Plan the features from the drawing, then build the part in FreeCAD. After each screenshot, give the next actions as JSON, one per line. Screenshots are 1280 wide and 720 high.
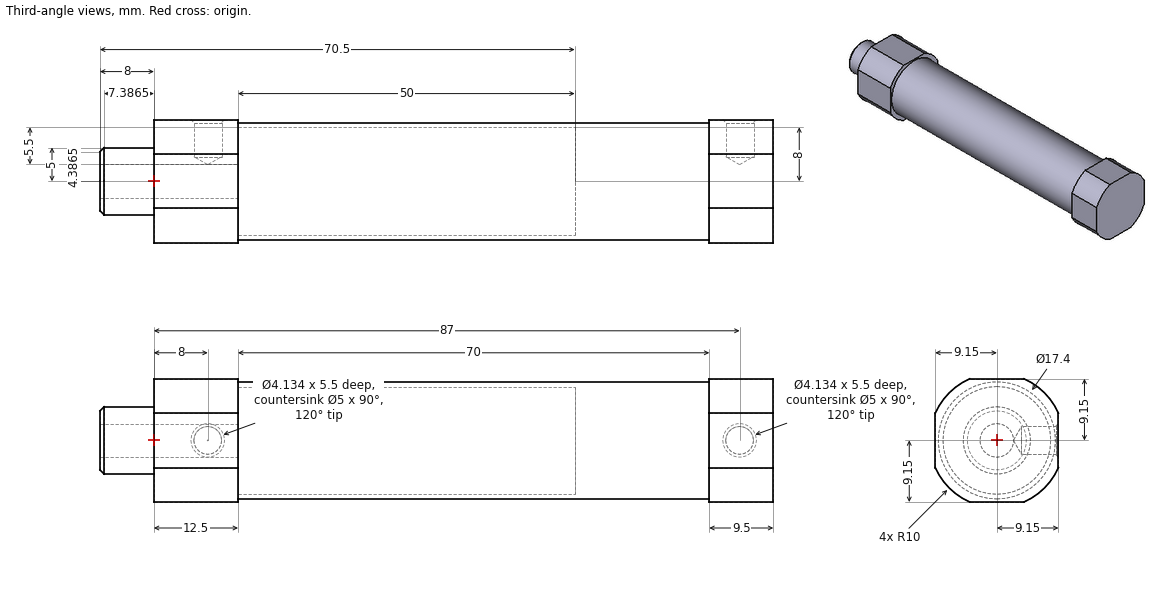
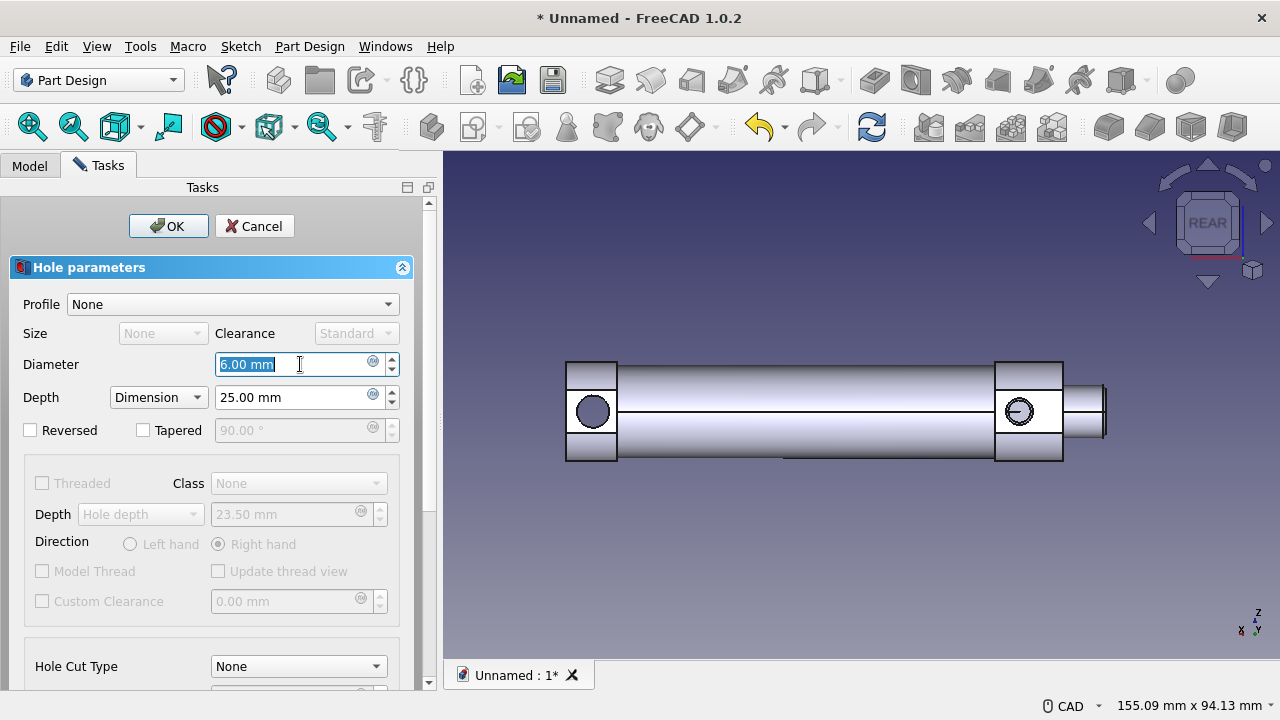
{"action": "type", "text": "4.134"}
{"action": "key", "text": "Tab"}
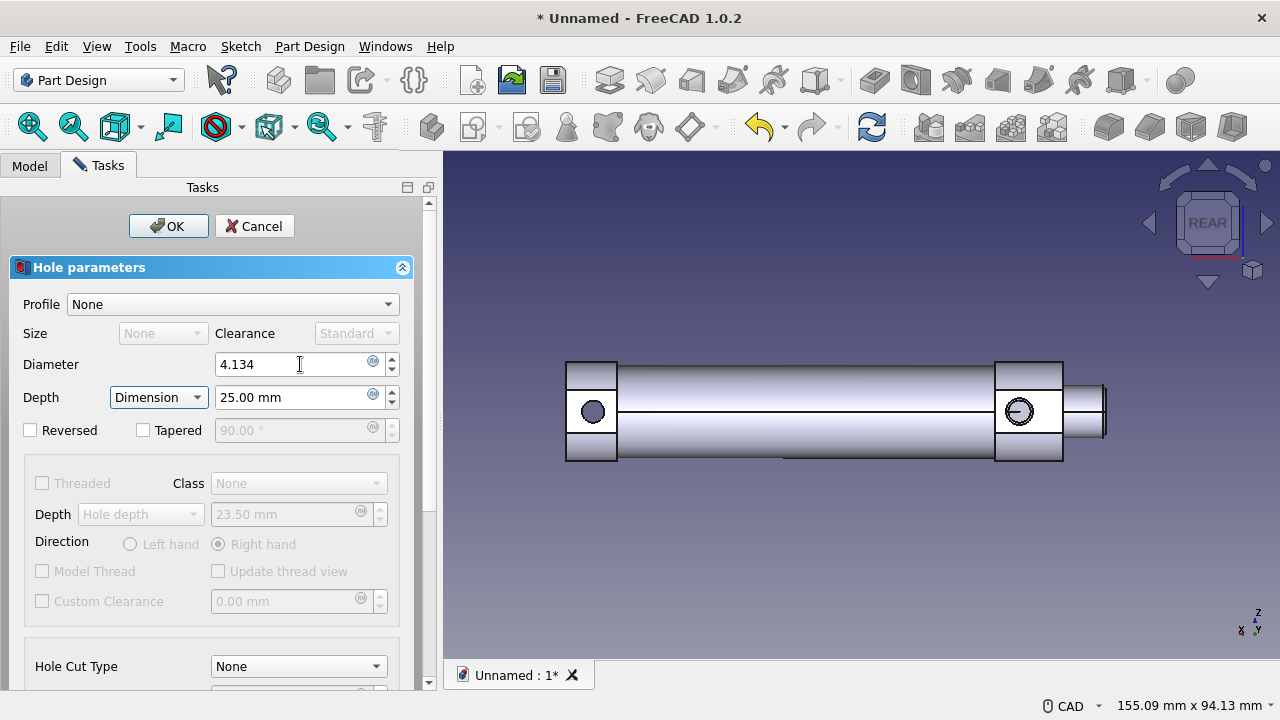
{"action": "triple_click", "coordinate": [300, 398]}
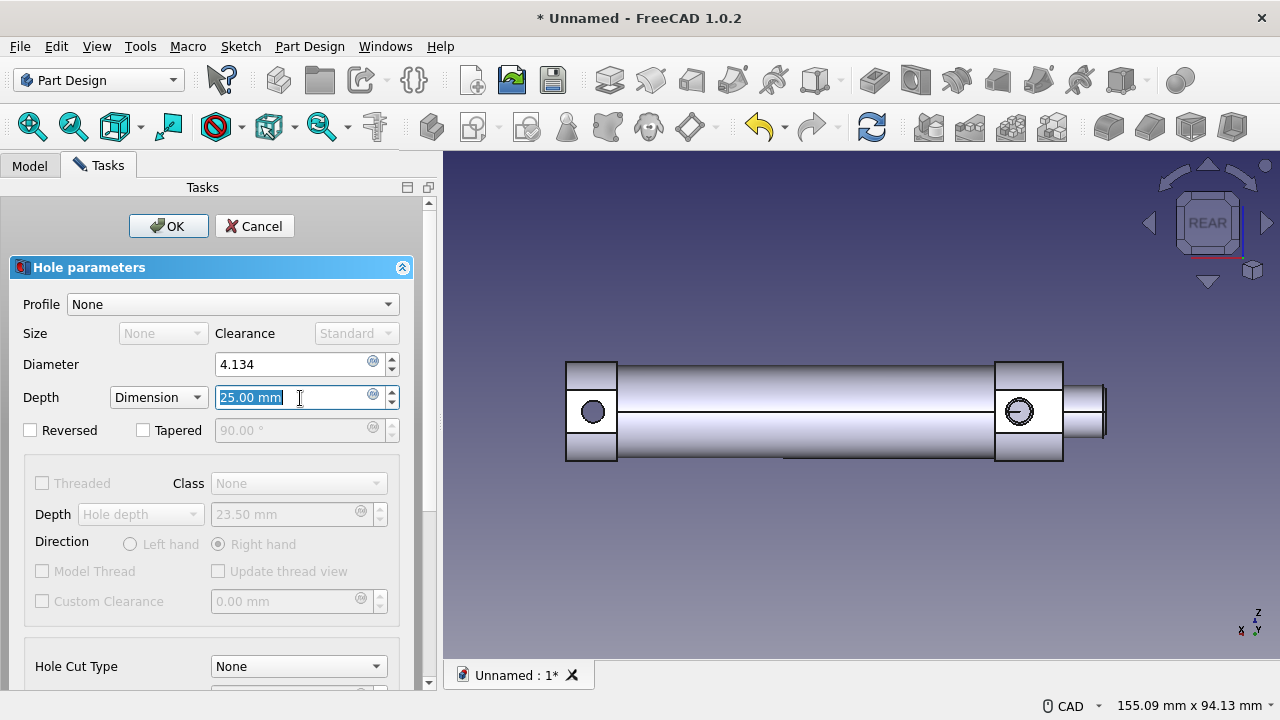
{"action": "type", "text": "5.5"}
{"action": "key", "text": "Tab"}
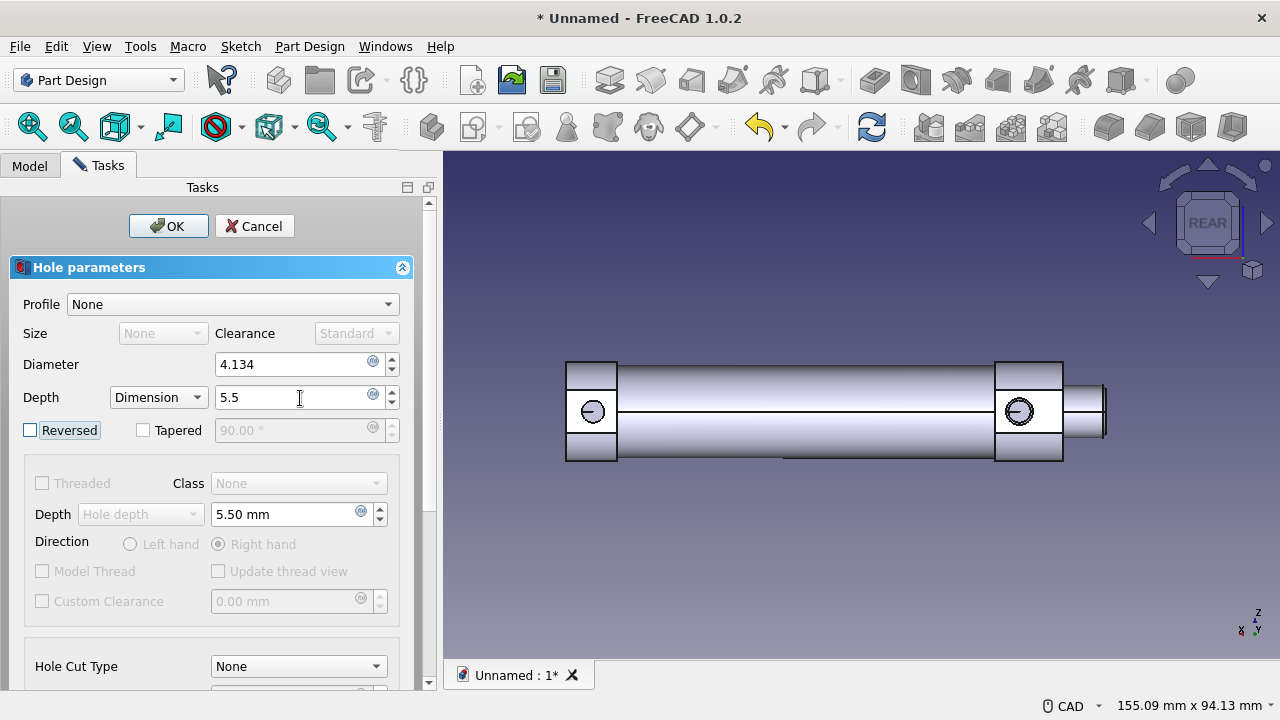
{"action": "left_click", "coordinate": [300, 666]}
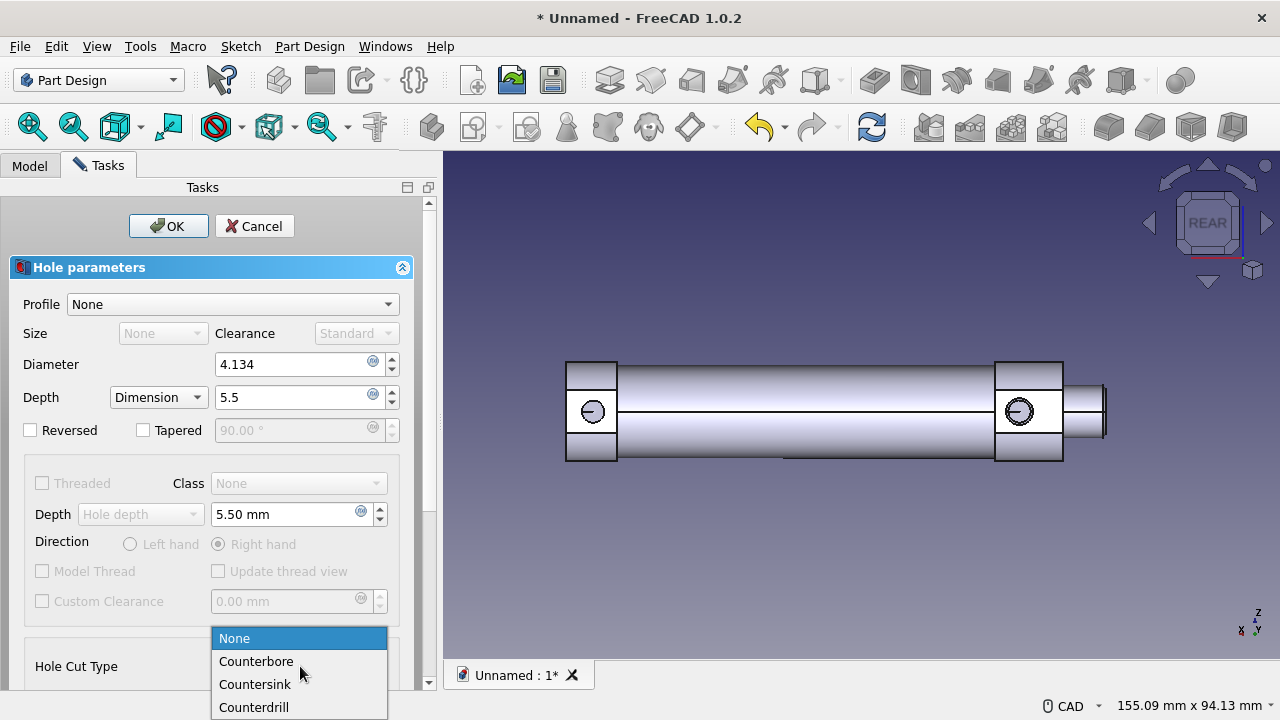
{"action": "left_click", "coordinate": [298, 684]}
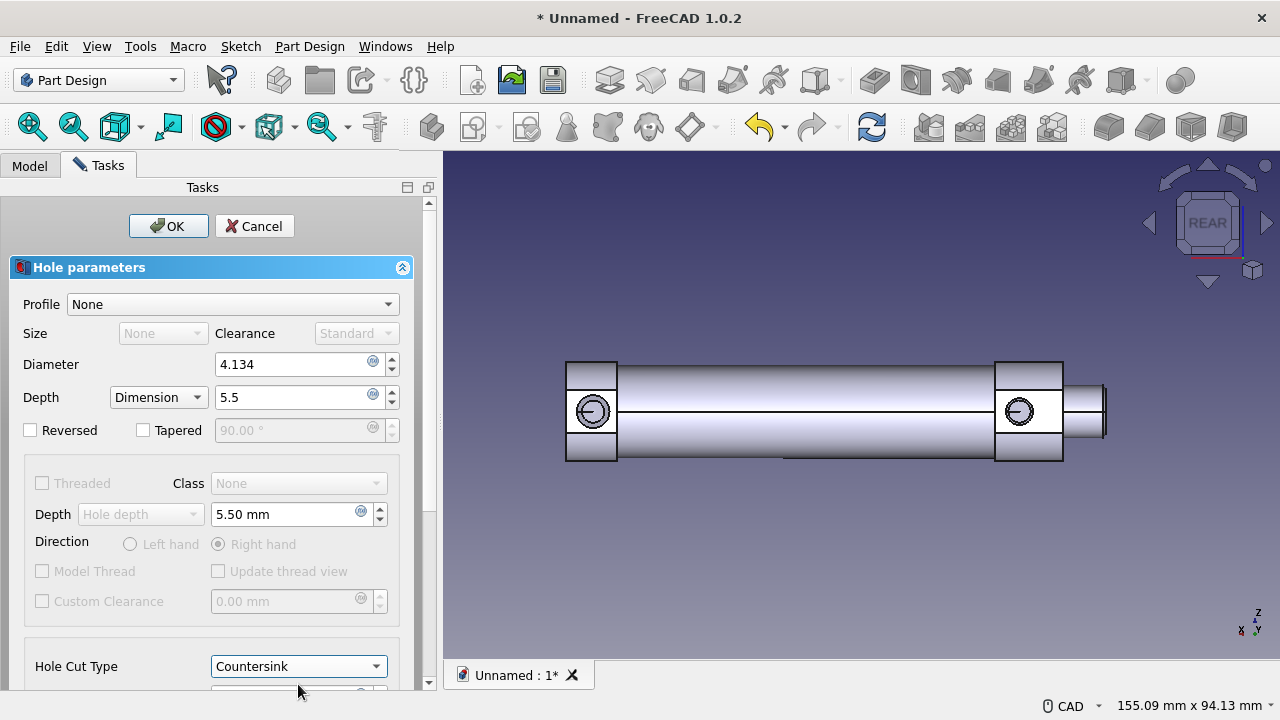
{"action": "scroll", "coordinate": [429, 444], "scroll_direction": "down", "scroll_amount": 2}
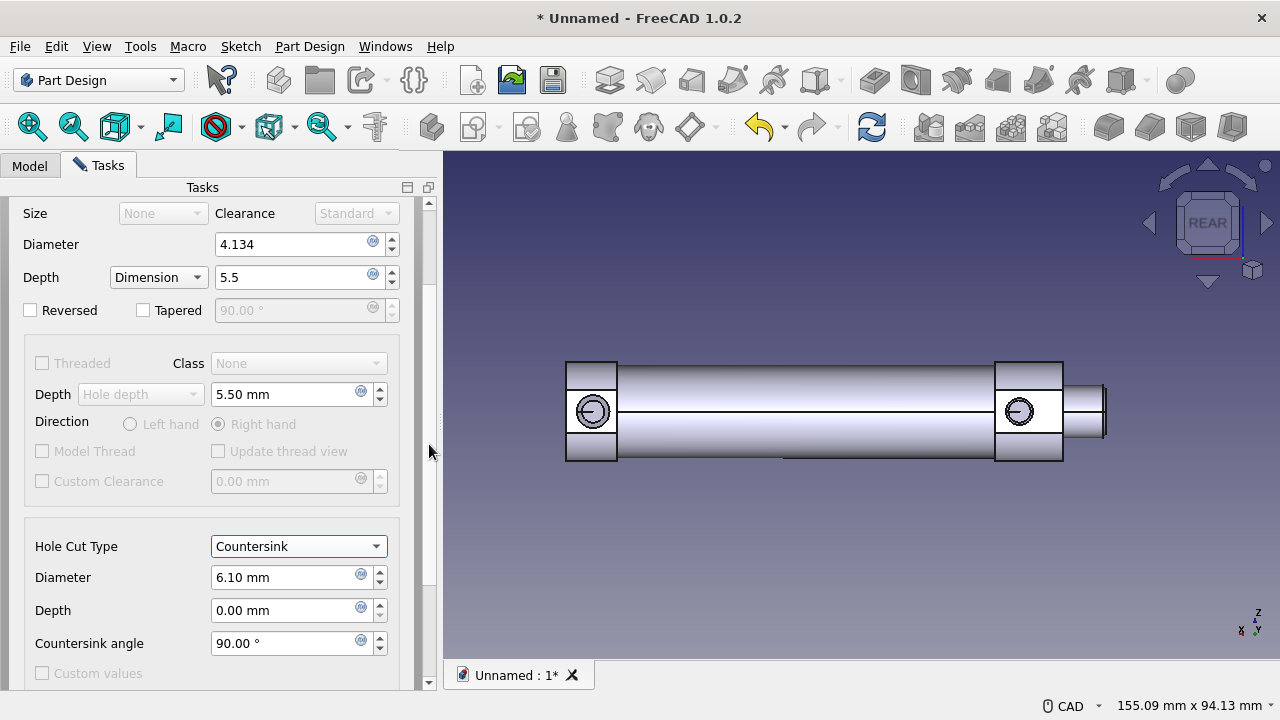
{"action": "triple_click", "coordinate": [292, 578]}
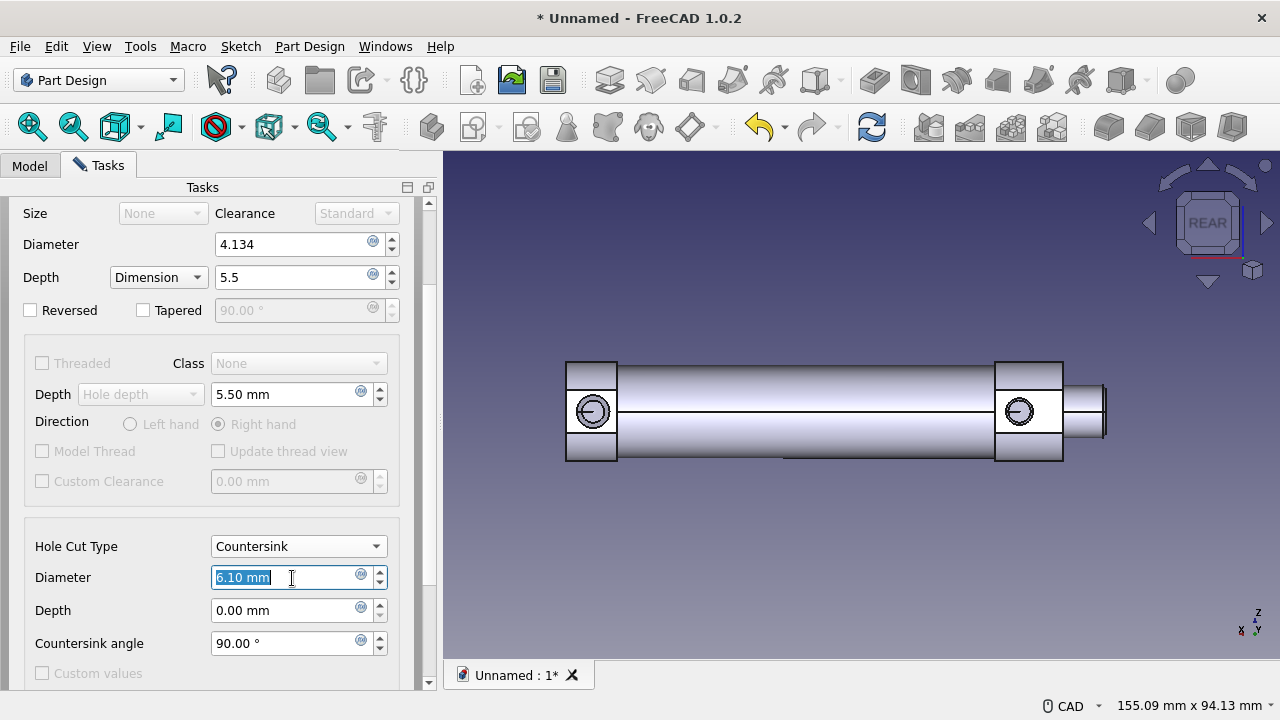
{"action": "type", "text": "5"}
{"action": "key", "text": "Tab"}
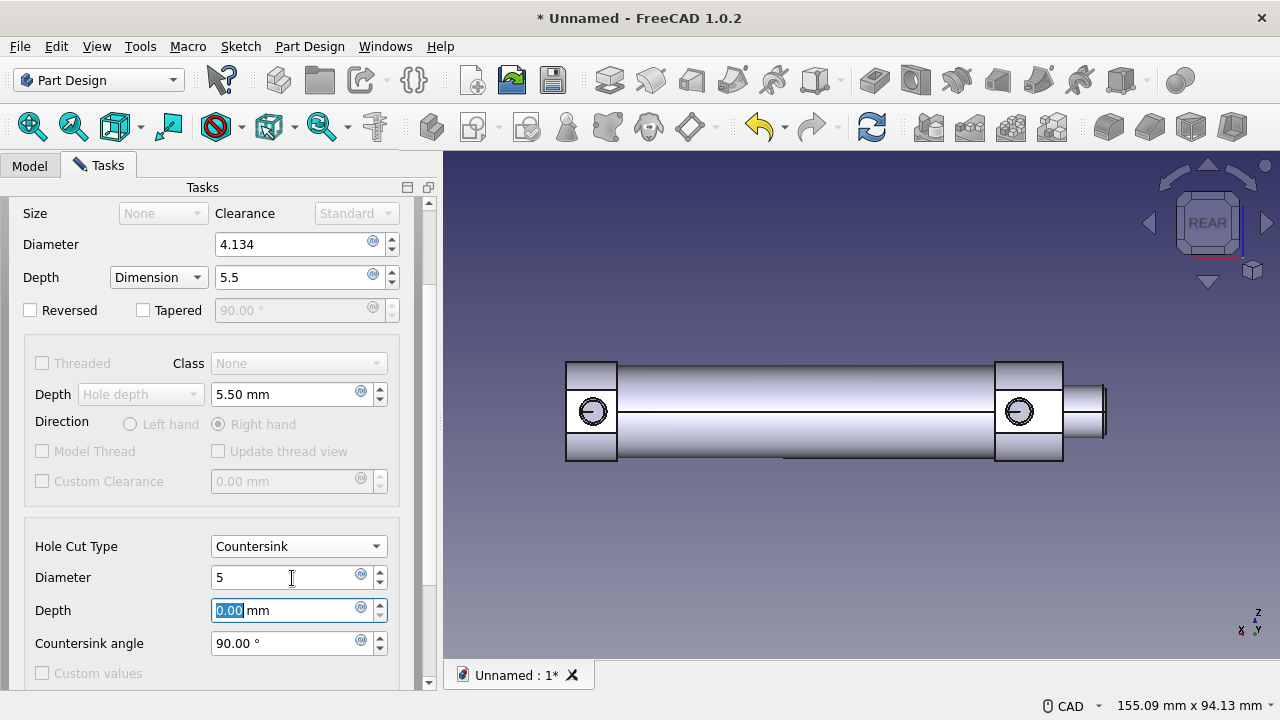
{"action": "scroll", "coordinate": [429, 444], "scroll_direction": "down", "scroll_amount": 3}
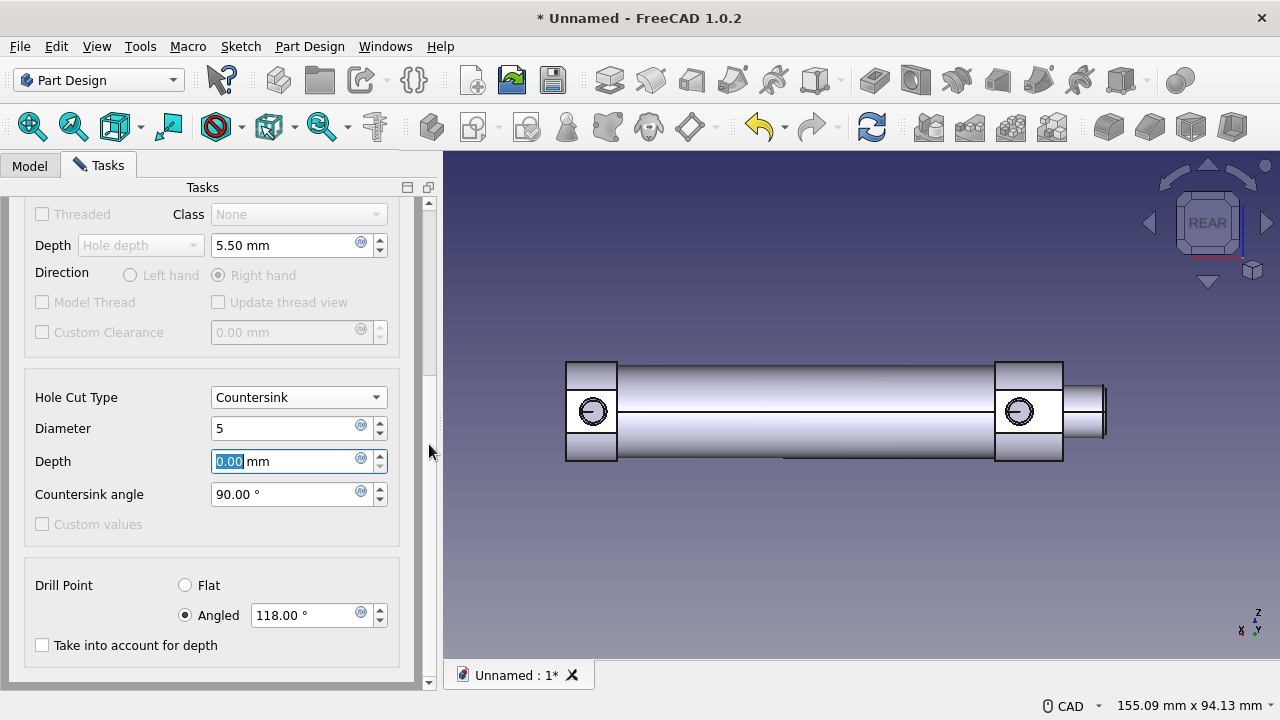
{"action": "triple_click", "coordinate": [312, 616]}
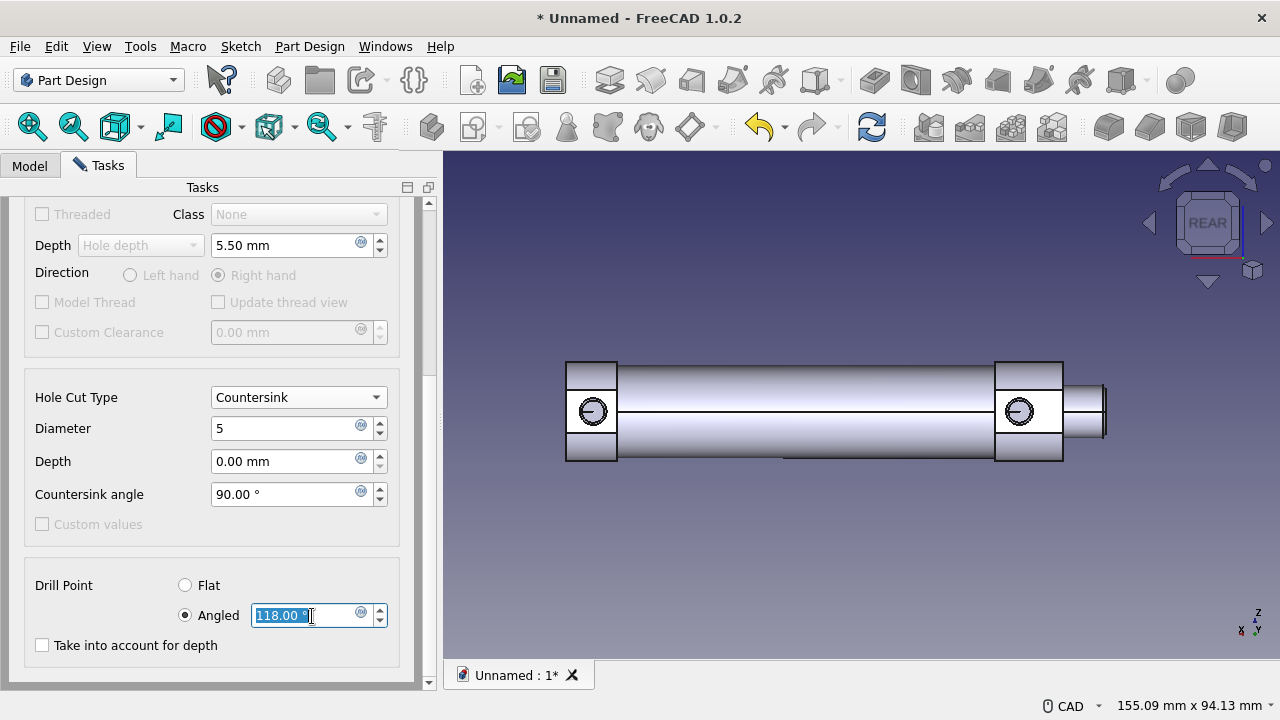
{"action": "type", "text": "120"}
{"action": "key", "text": "Tab"}